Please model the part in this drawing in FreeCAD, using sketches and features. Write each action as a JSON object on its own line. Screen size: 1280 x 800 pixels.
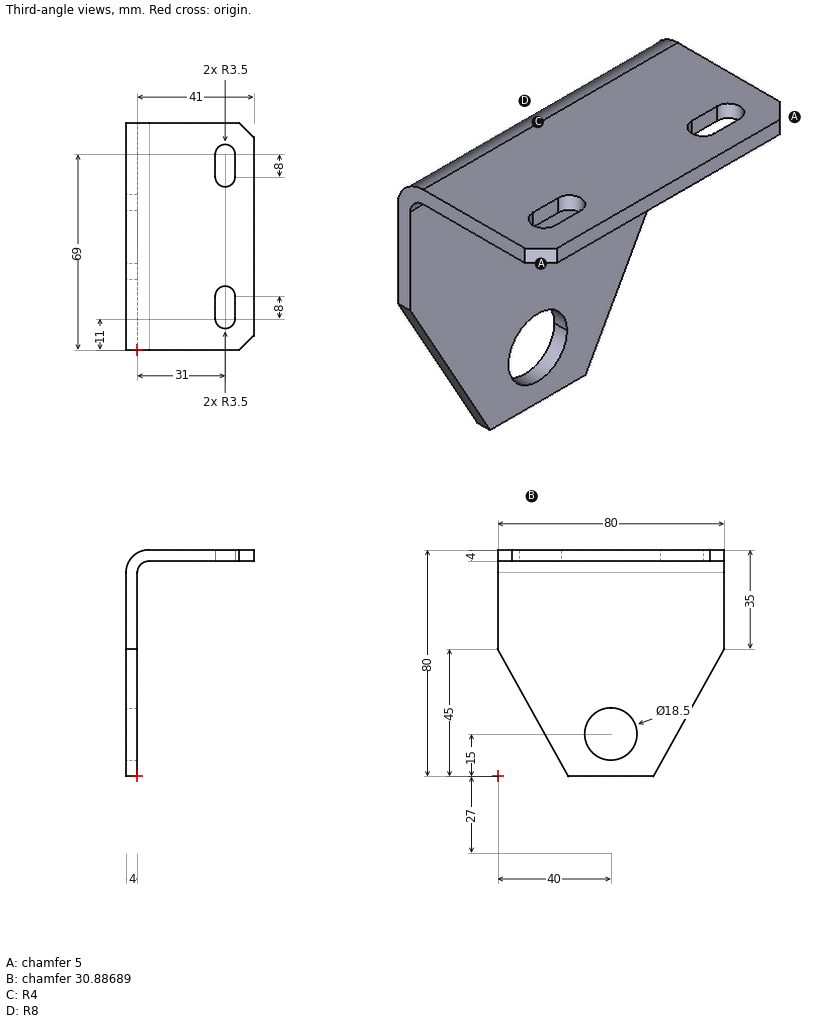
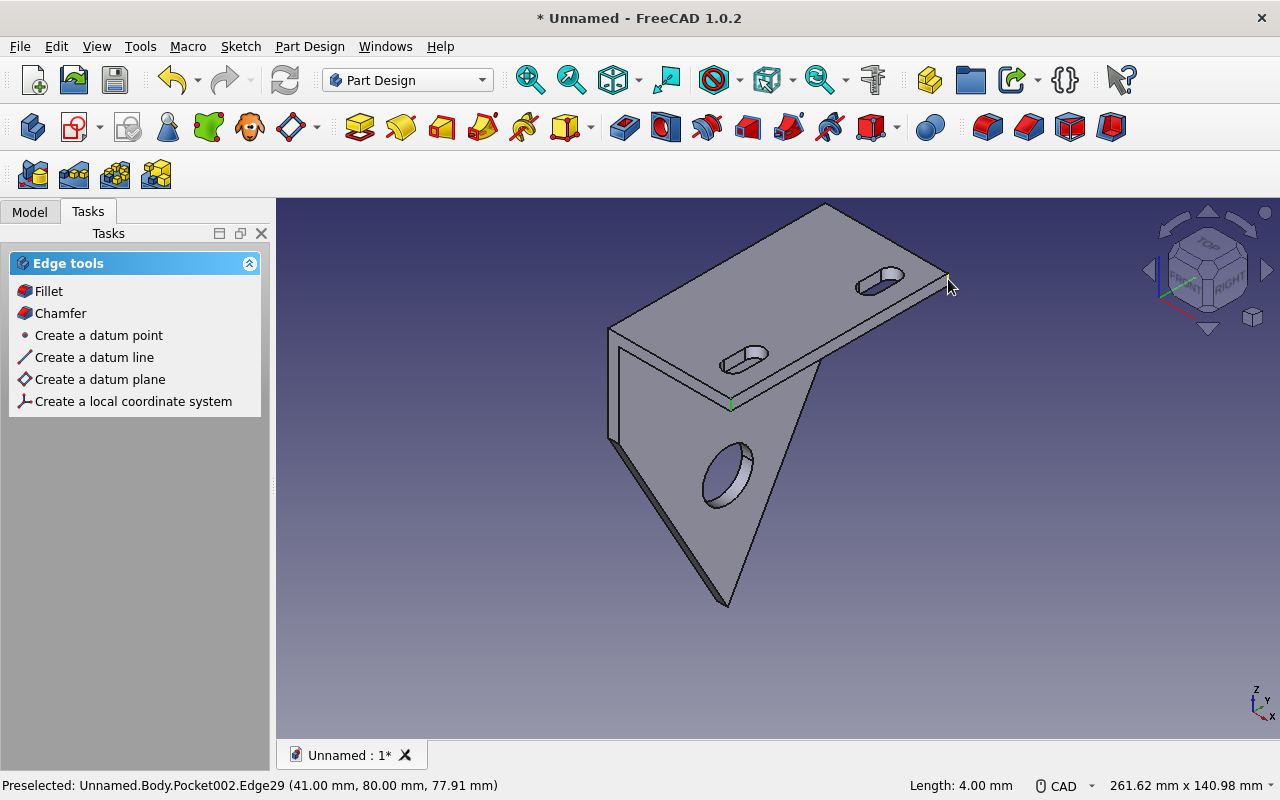
{"action": "key", "text": "2"}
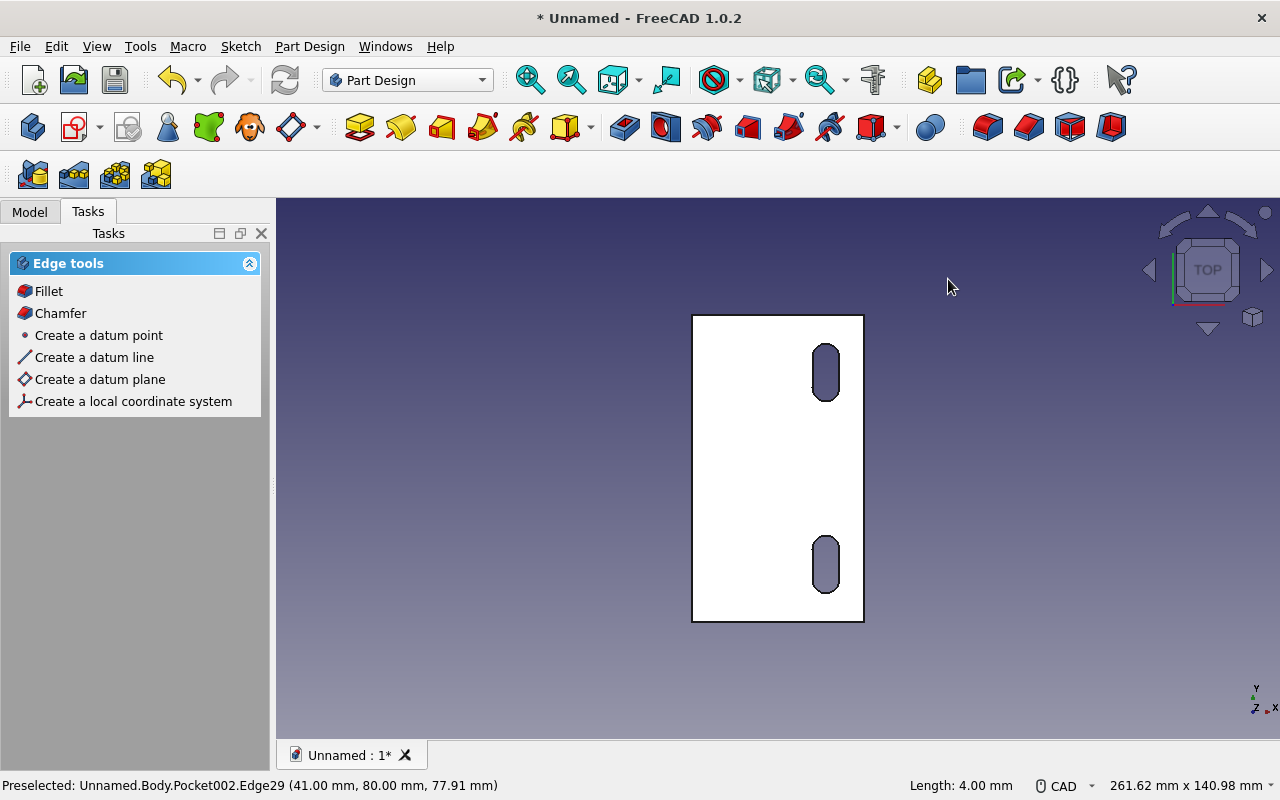
{"action": "scroll", "coordinate": [864, 314], "scroll_direction": "up", "scroll_amount": 5}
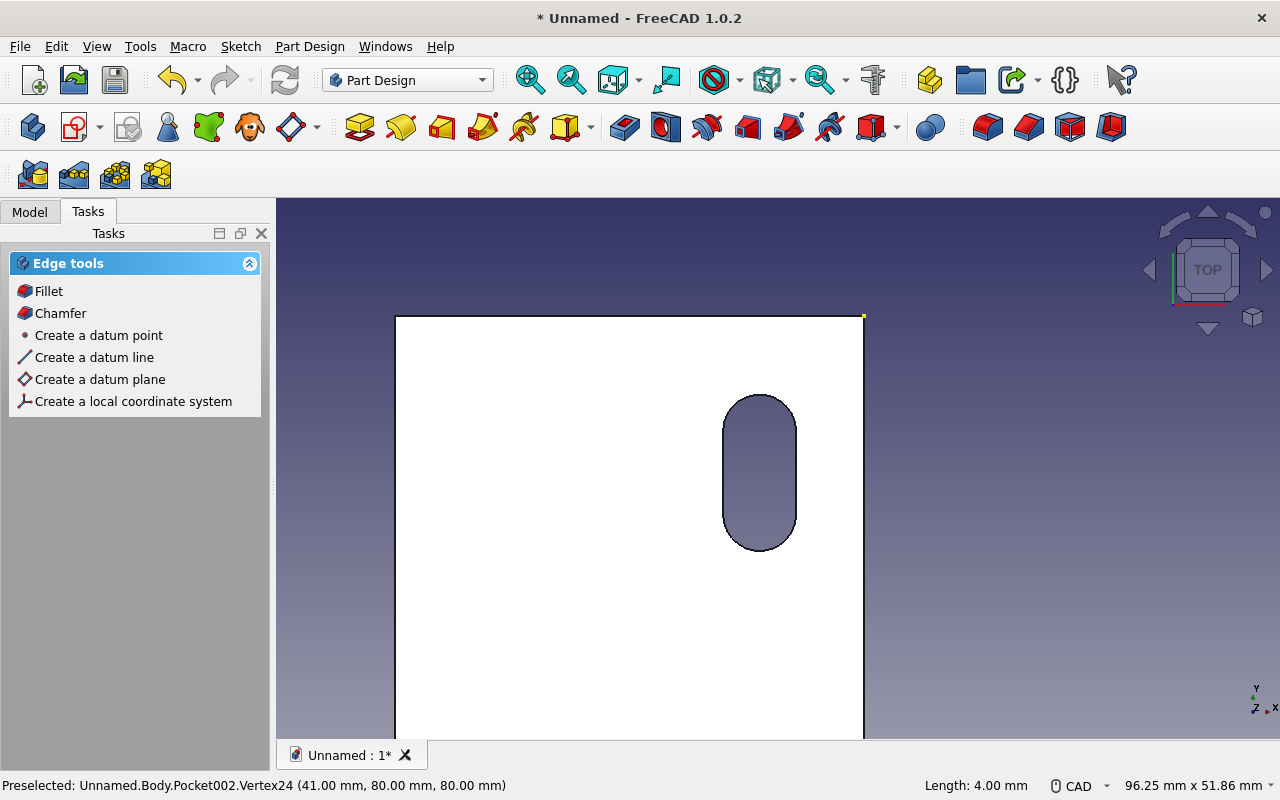
{"action": "key", "text": "v f"}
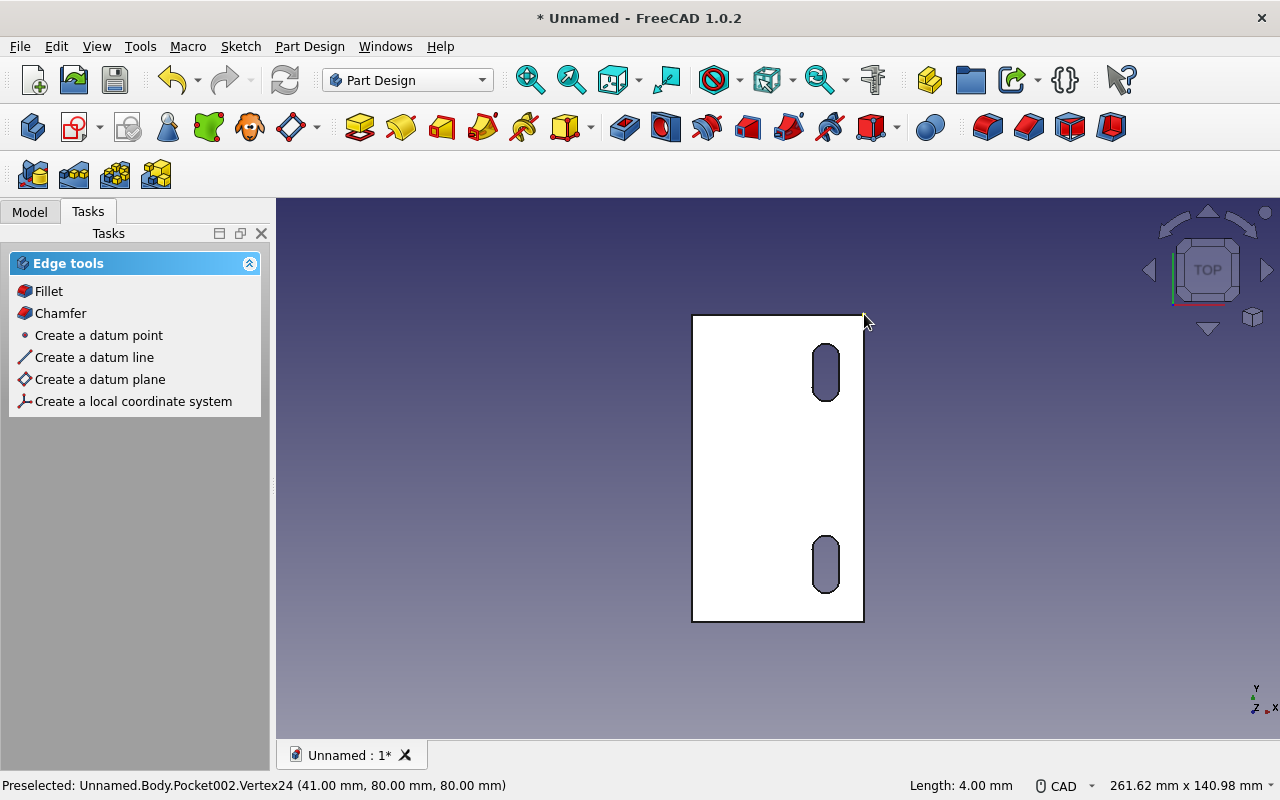
{"action": "key", "text": "0"}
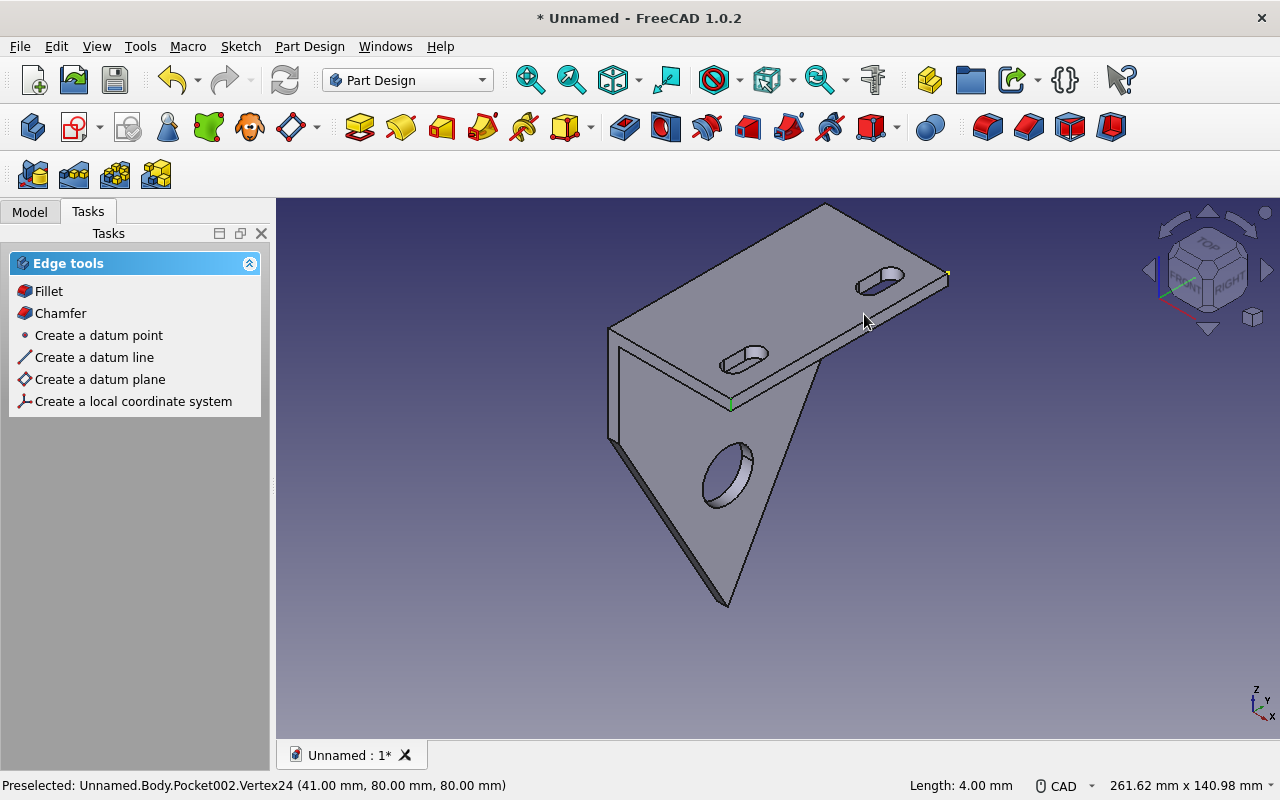
{"action": "scroll", "coordinate": [948, 279], "scroll_direction": "up", "scroll_amount": 5}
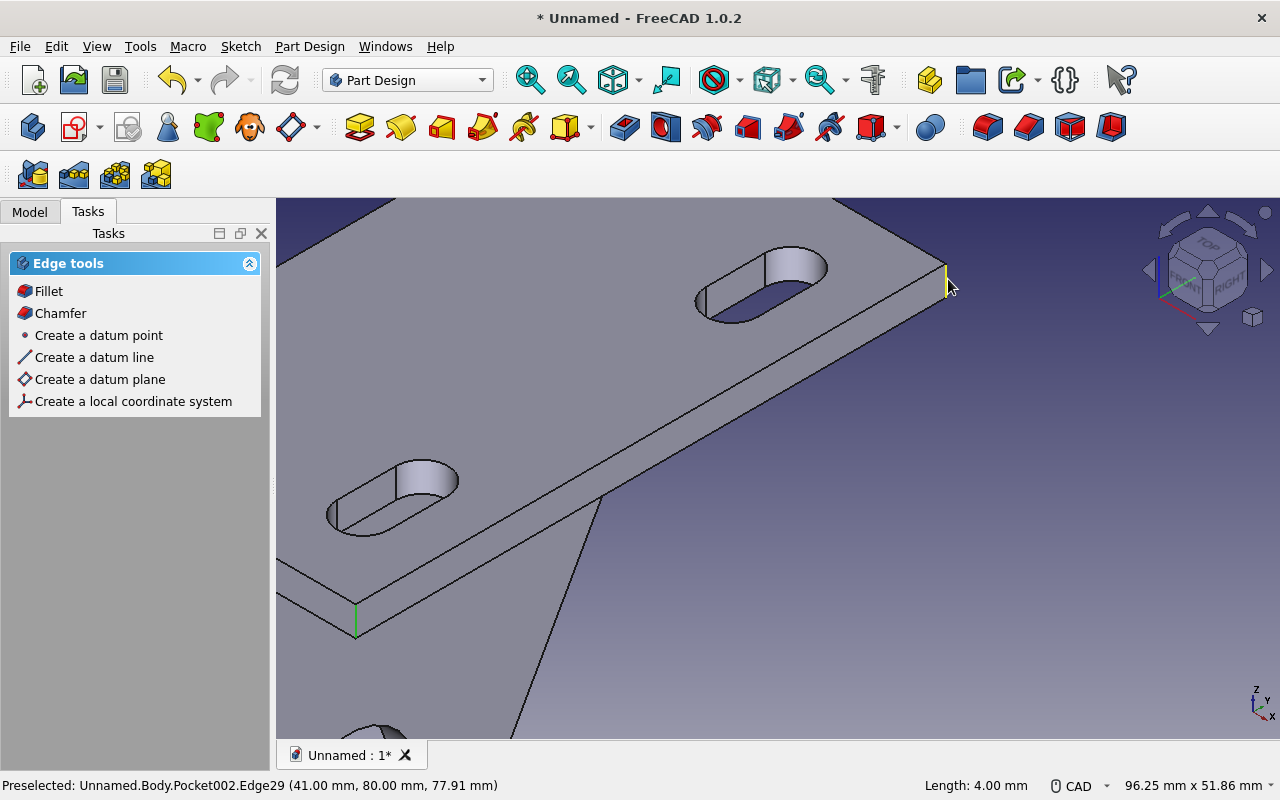
{"action": "left_click", "coordinate": [531, 80]}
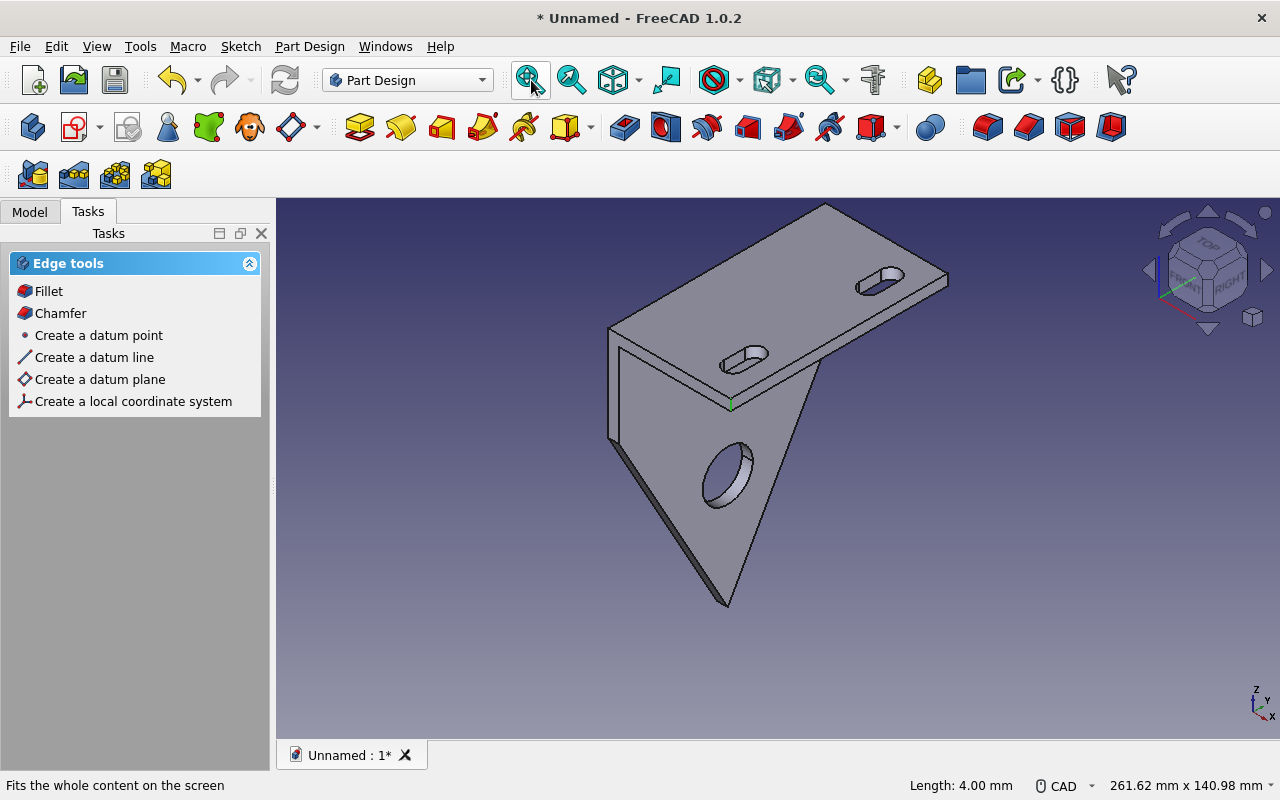
{"action": "key", "text": "1"}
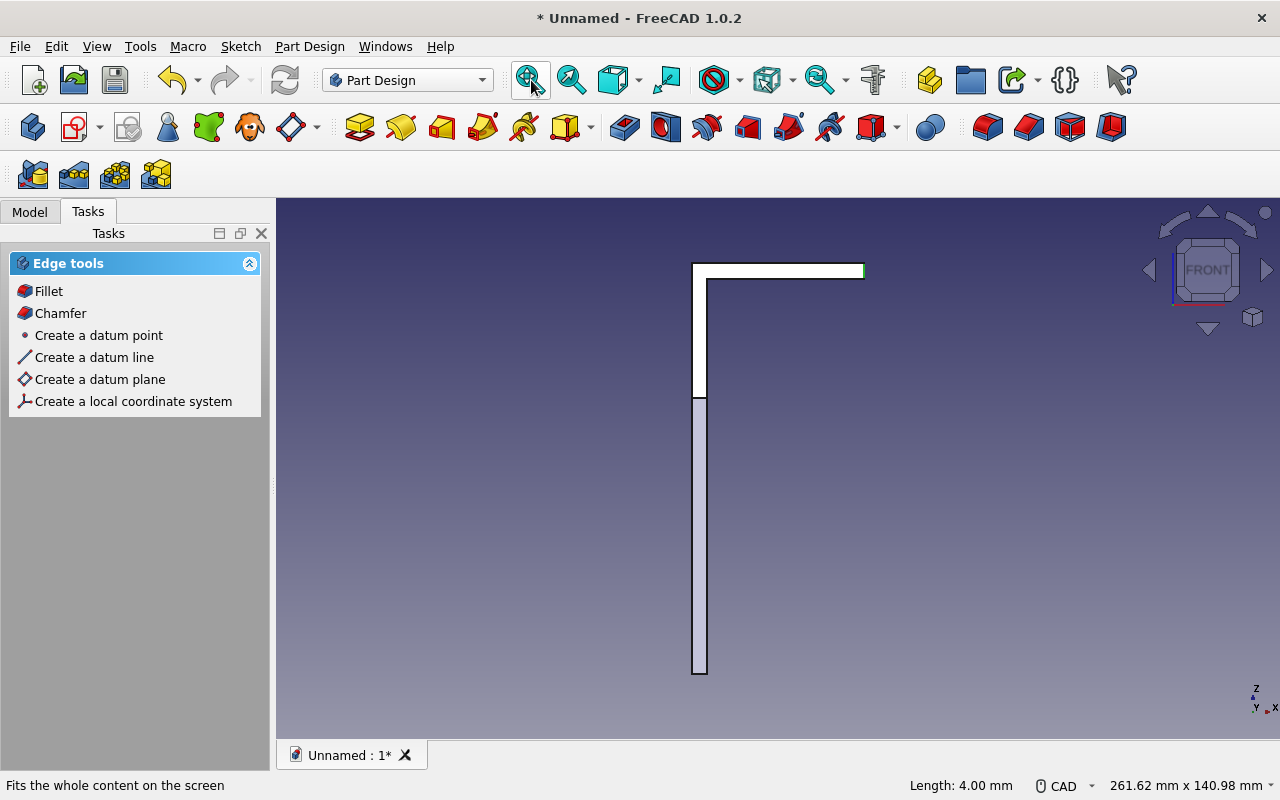
{"action": "scroll", "coordinate": [864, 270], "scroll_direction": "up", "scroll_amount": 5}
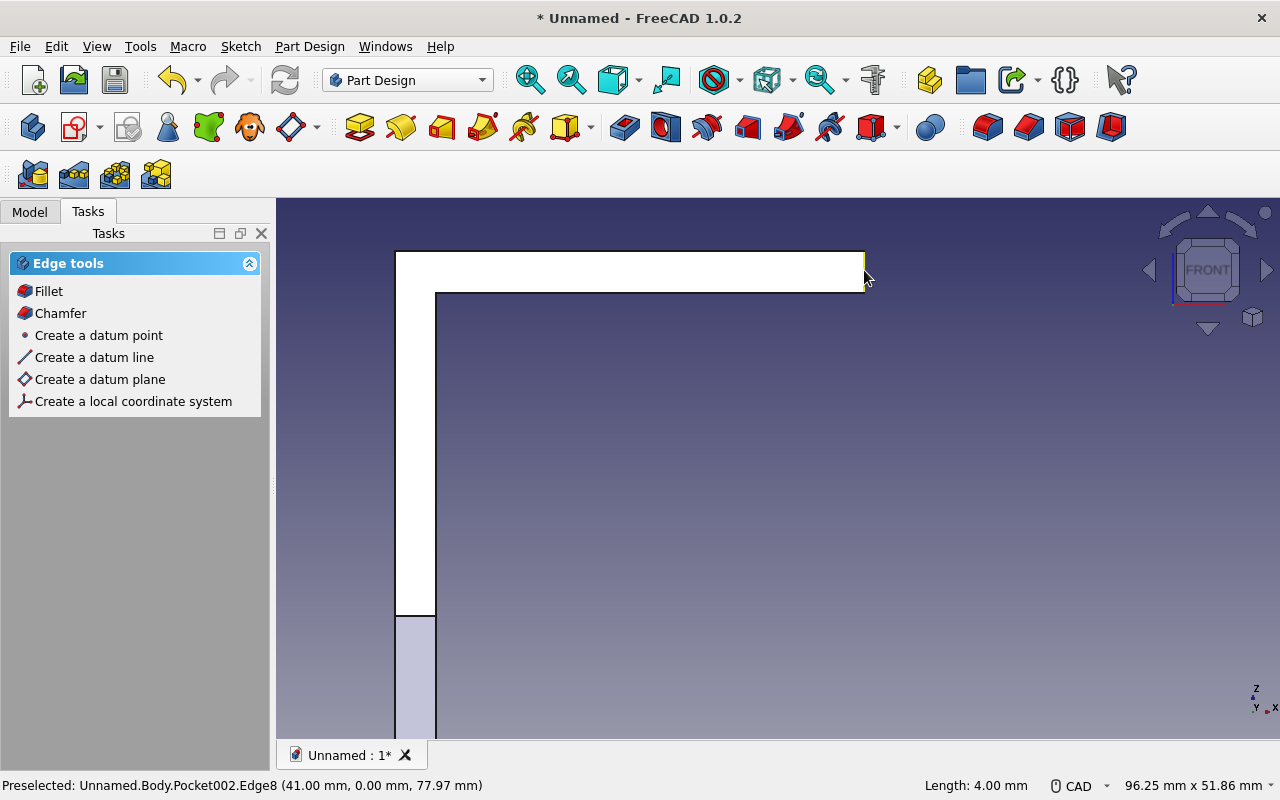
{"action": "left_click", "coordinate": [531, 80]}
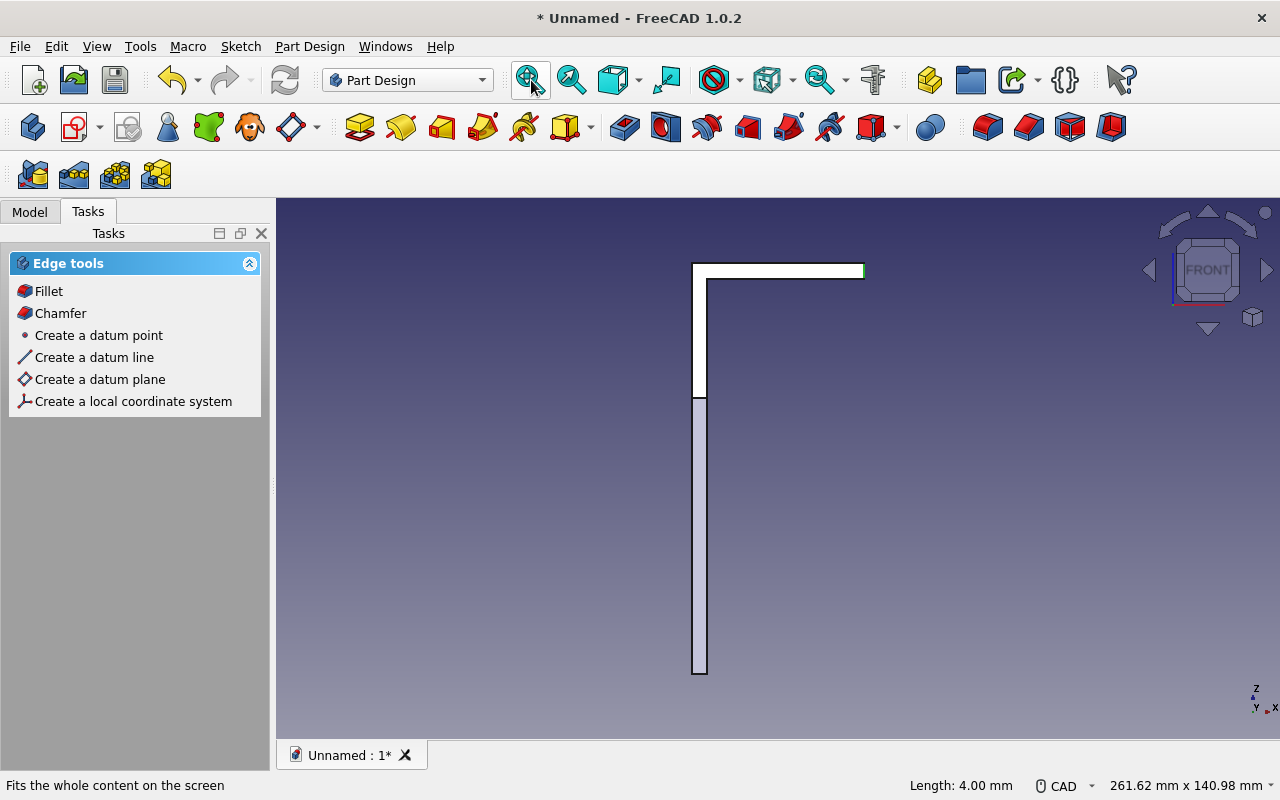
{"action": "key", "text": "3"}